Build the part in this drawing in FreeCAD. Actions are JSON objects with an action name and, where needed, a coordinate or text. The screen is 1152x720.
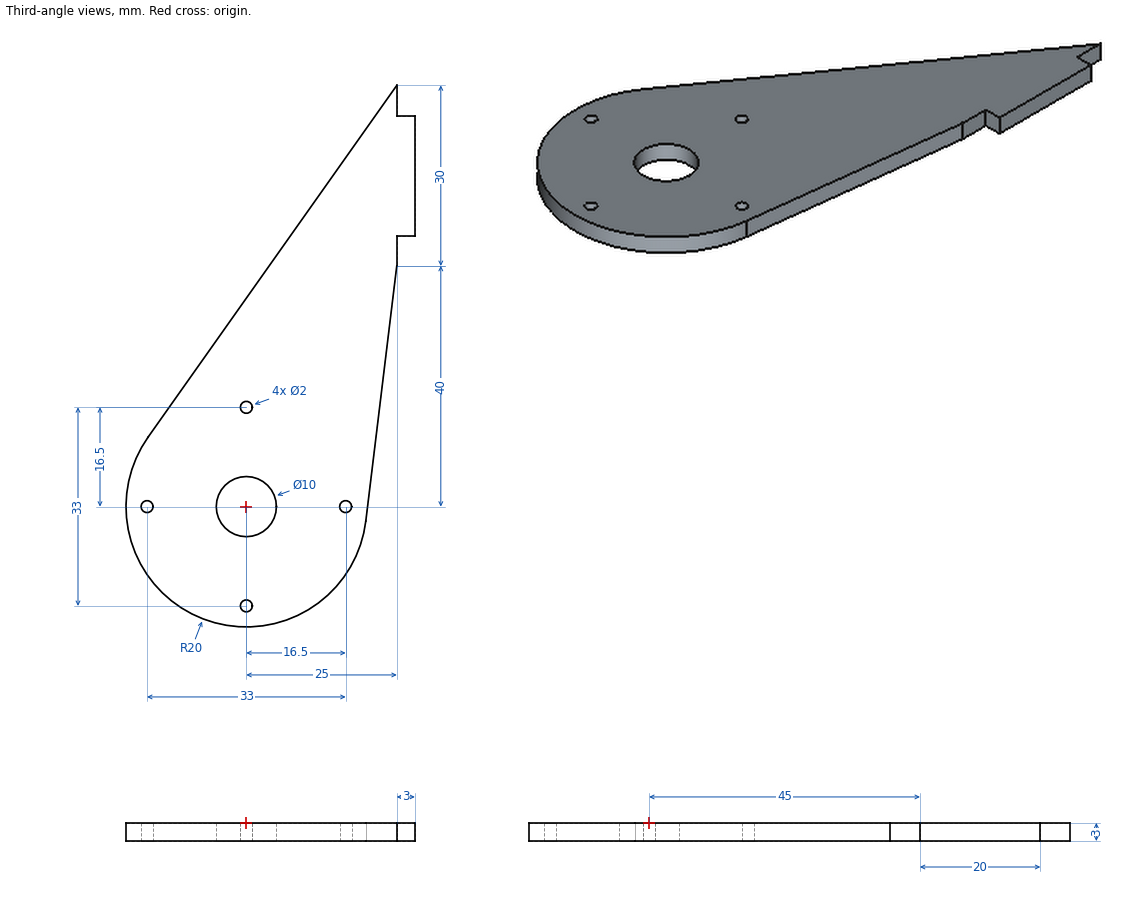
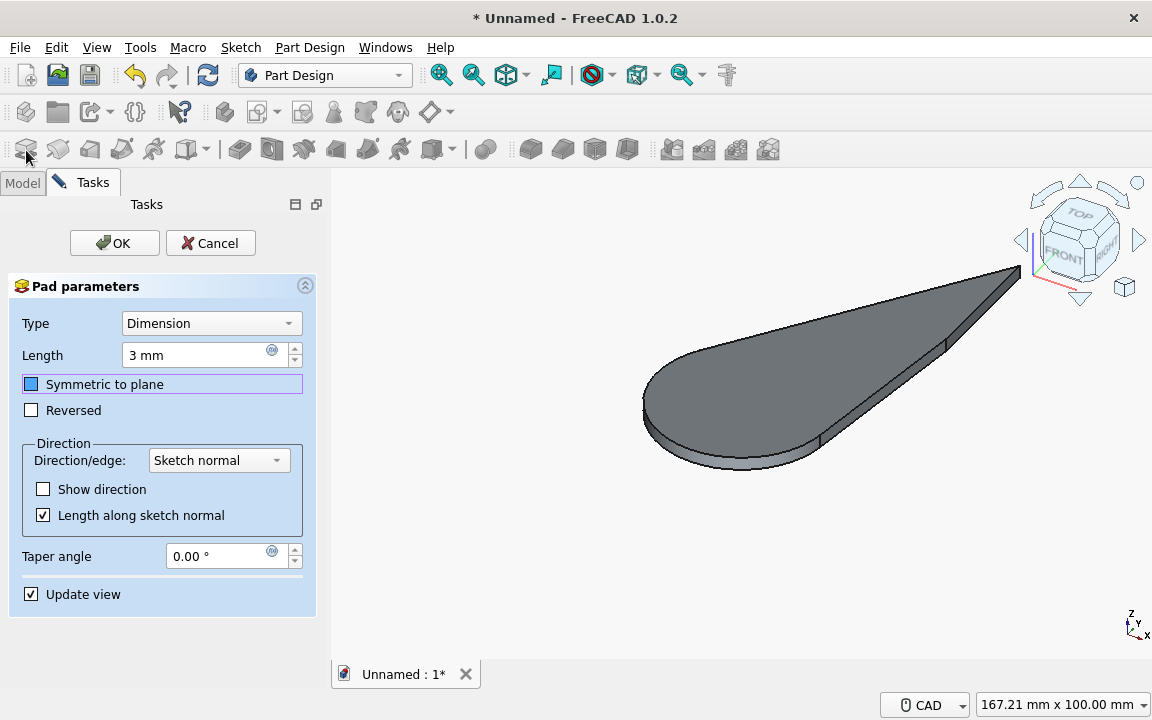
{"action": "left_click", "coordinate": [30, 410]}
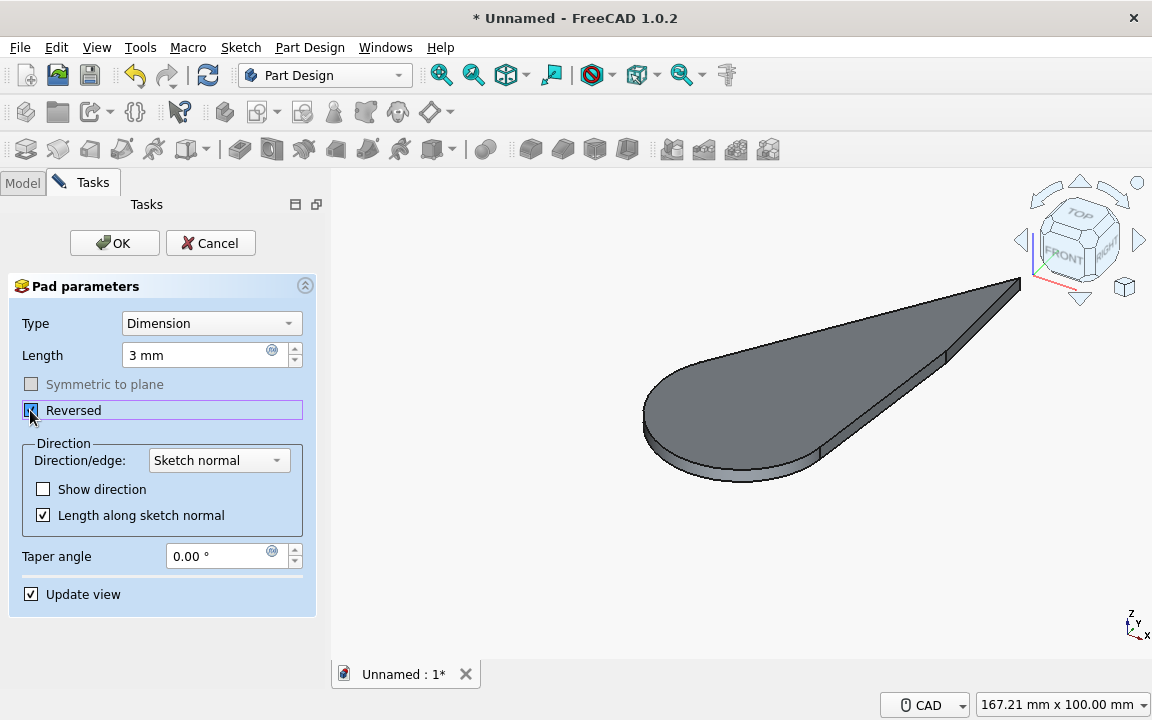
{"action": "left_click", "coordinate": [115, 243]}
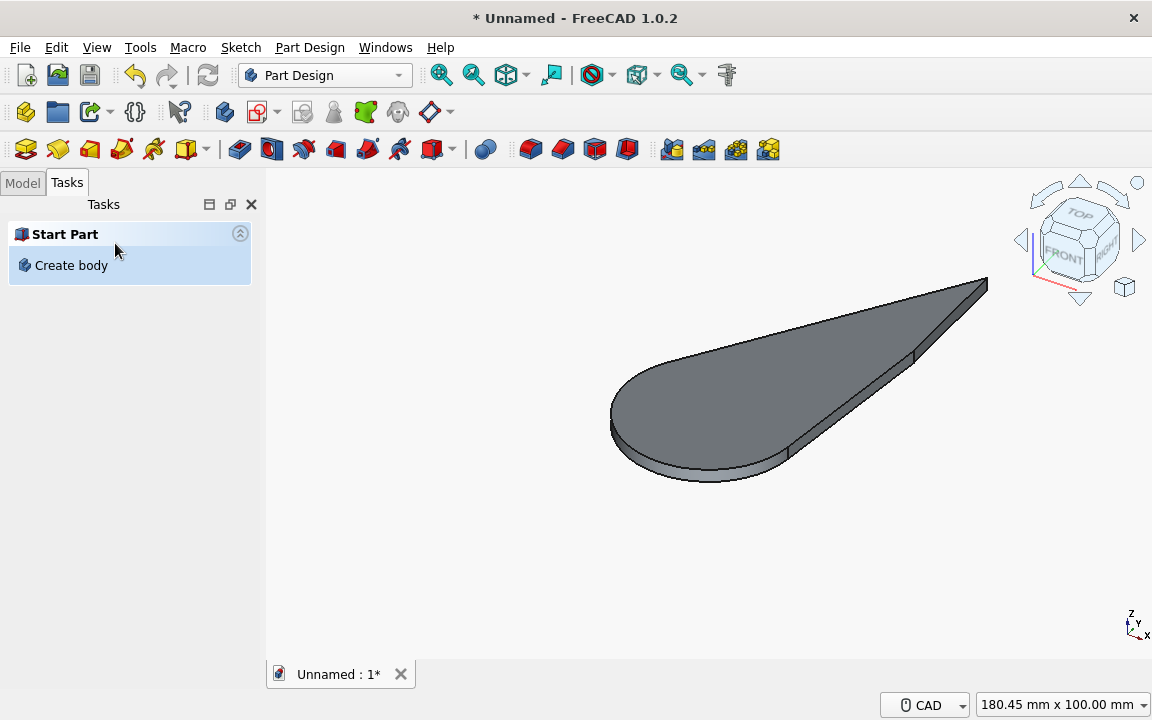
{"action": "left_click", "coordinate": [718, 418]}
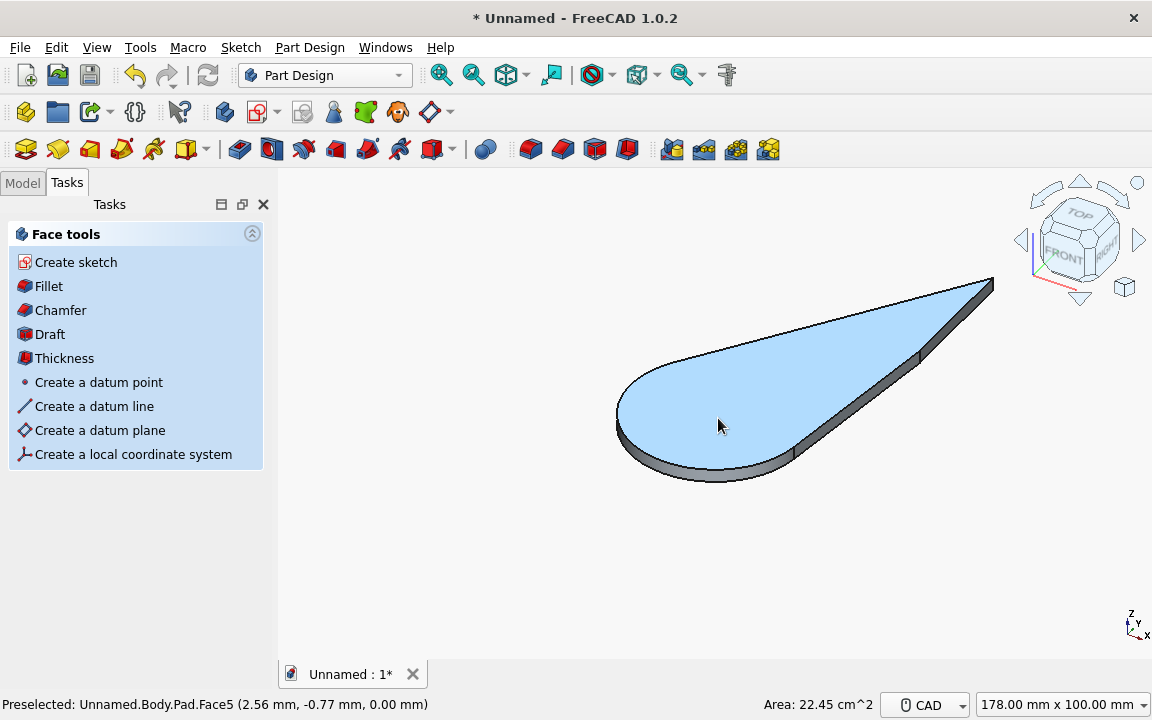
{"action": "left_click", "coordinate": [258, 112]}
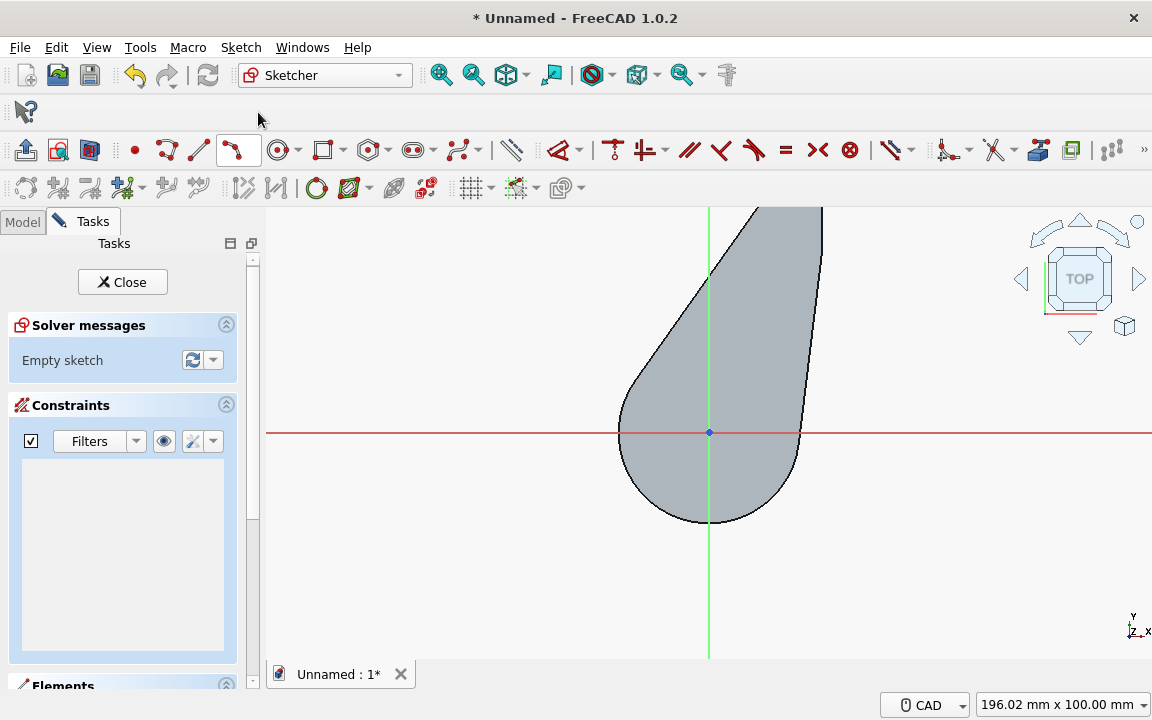
{"action": "scroll", "coordinate": [723, 433], "scroll_direction": "up", "scroll_amount": 9}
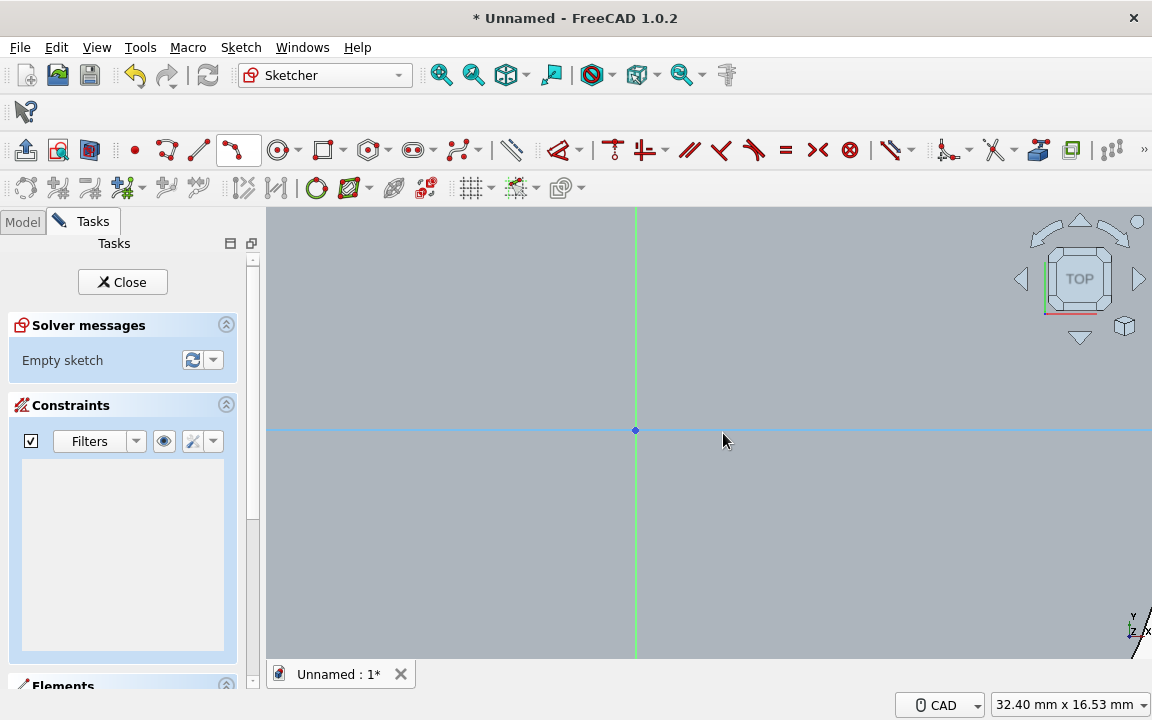
{"action": "left_click", "coordinate": [278, 150]}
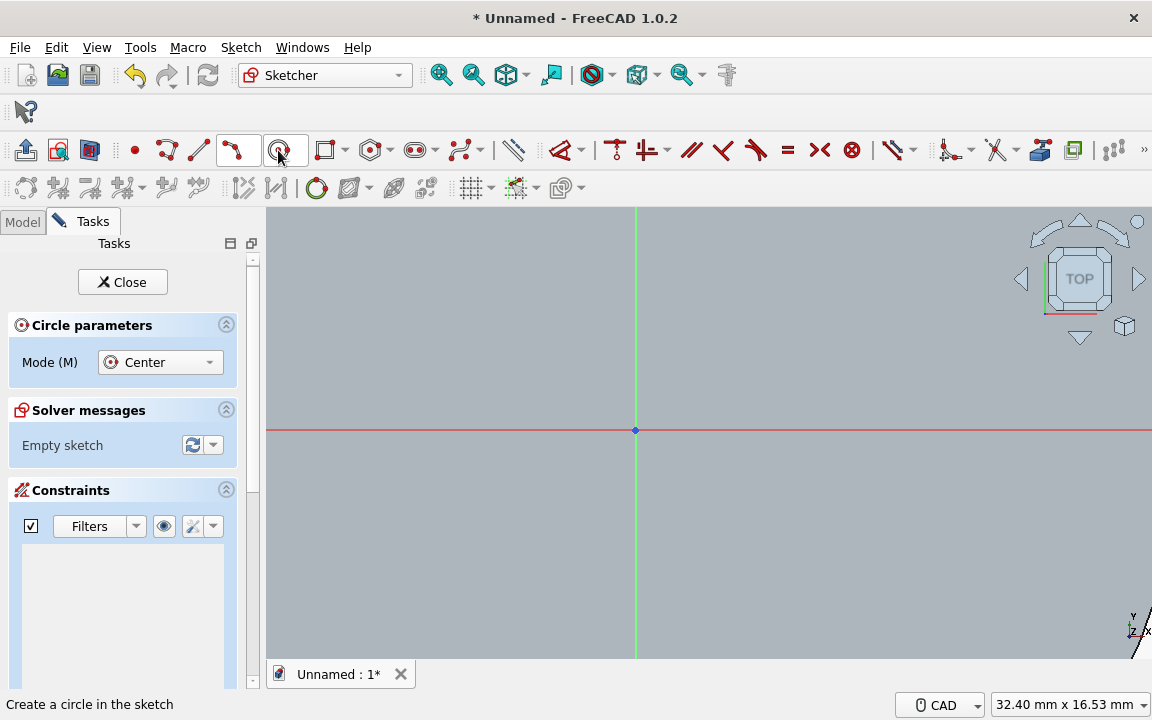
{"action": "left_click", "coordinate": [636, 430]}
{"action": "left_click", "coordinate": [732, 334]}
{"action": "key", "text": "Escape"}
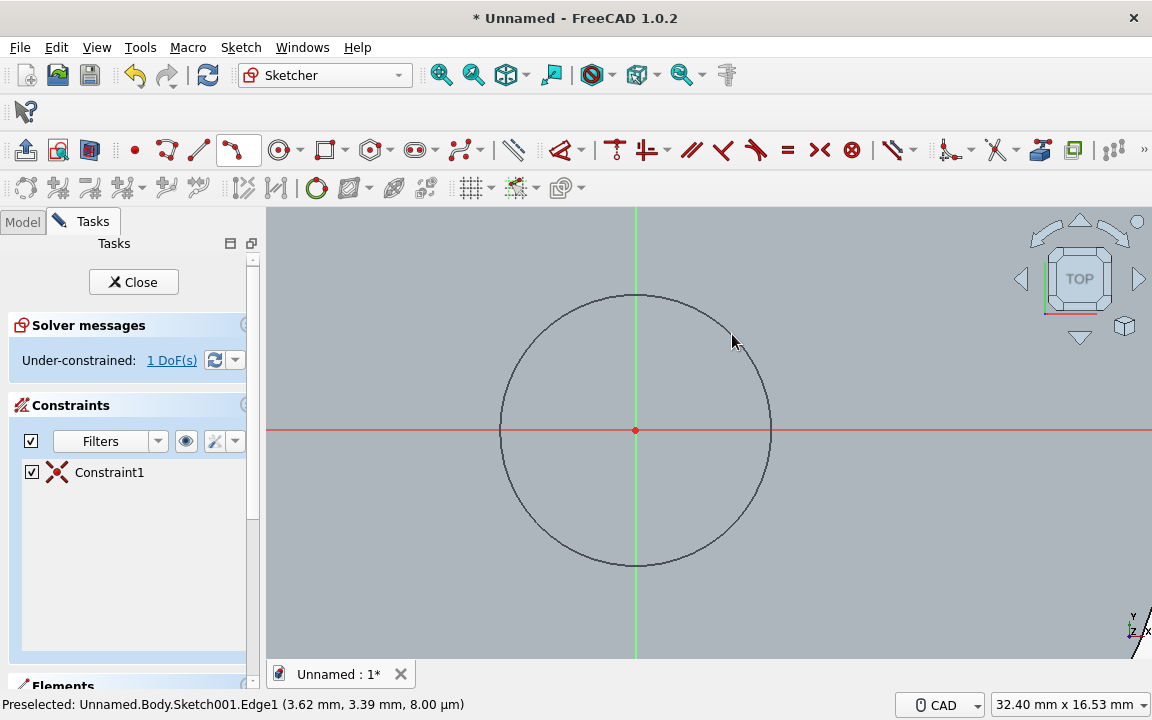
{"action": "left_click", "coordinate": [560, 150]}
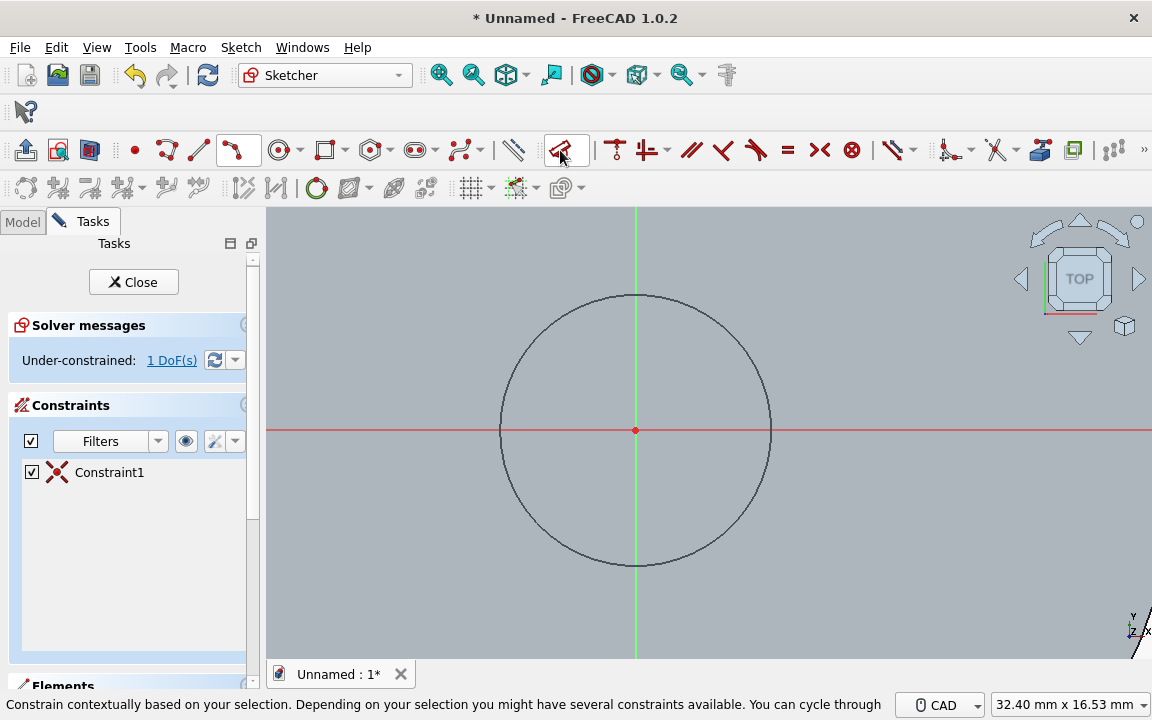
{"action": "left_click", "coordinate": [731, 334]}
{"action": "left_click", "coordinate": [753, 311]}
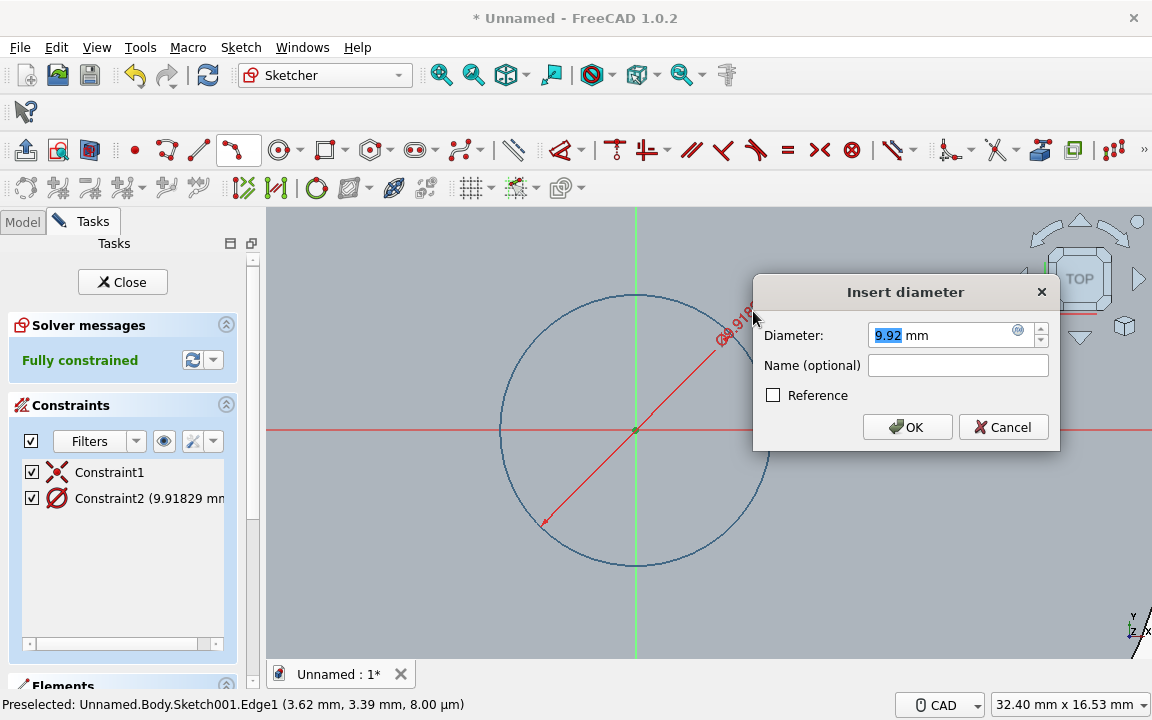
{"action": "type", "text": "10"}
{"action": "key", "text": "Return"}
{"action": "key", "text": "Escape"}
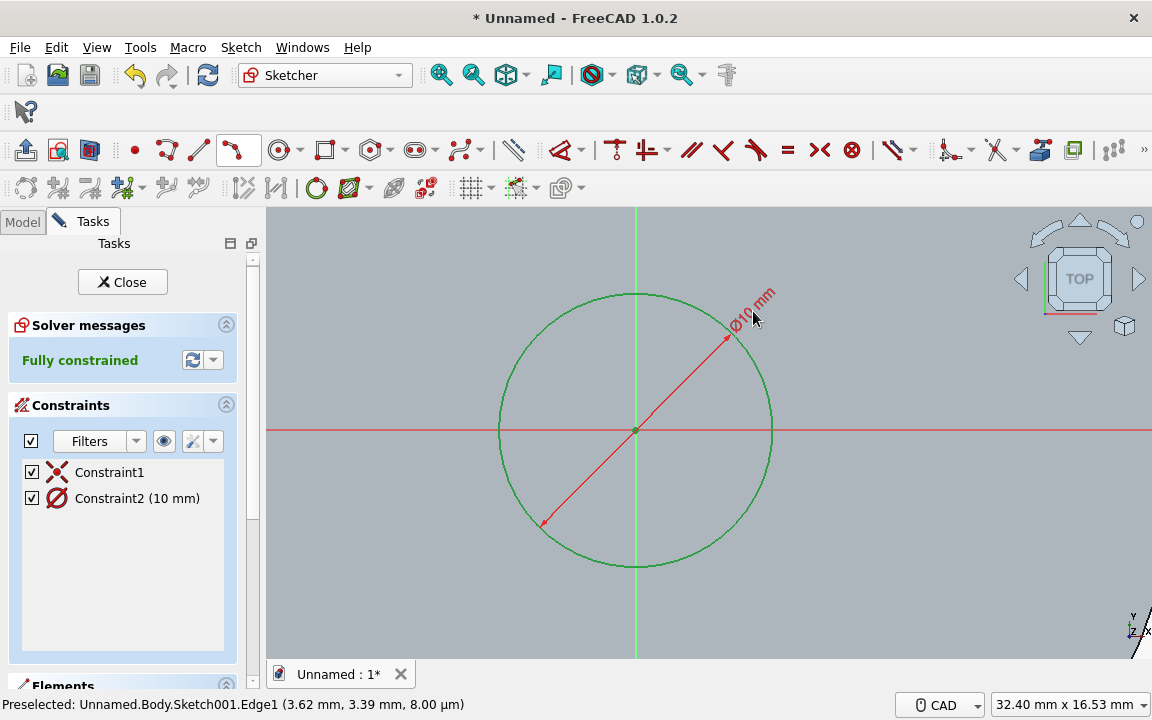
{"action": "left_click", "coordinate": [123, 282]}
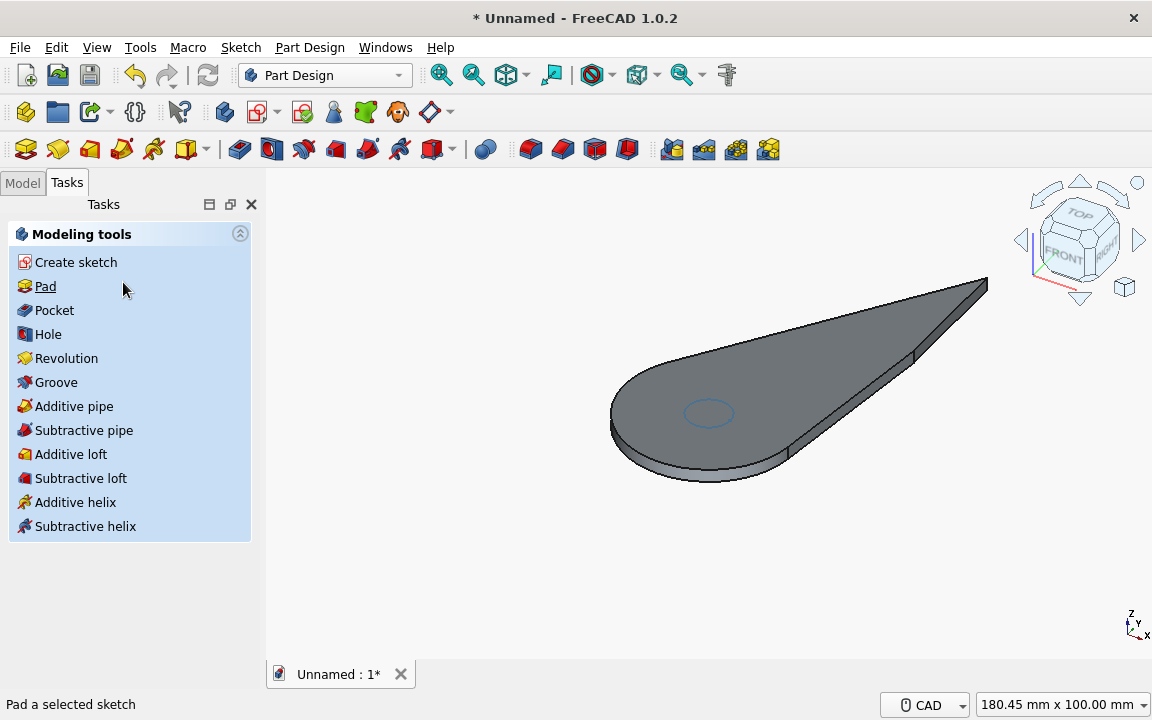
{"action": "left_click", "coordinate": [240, 150]}